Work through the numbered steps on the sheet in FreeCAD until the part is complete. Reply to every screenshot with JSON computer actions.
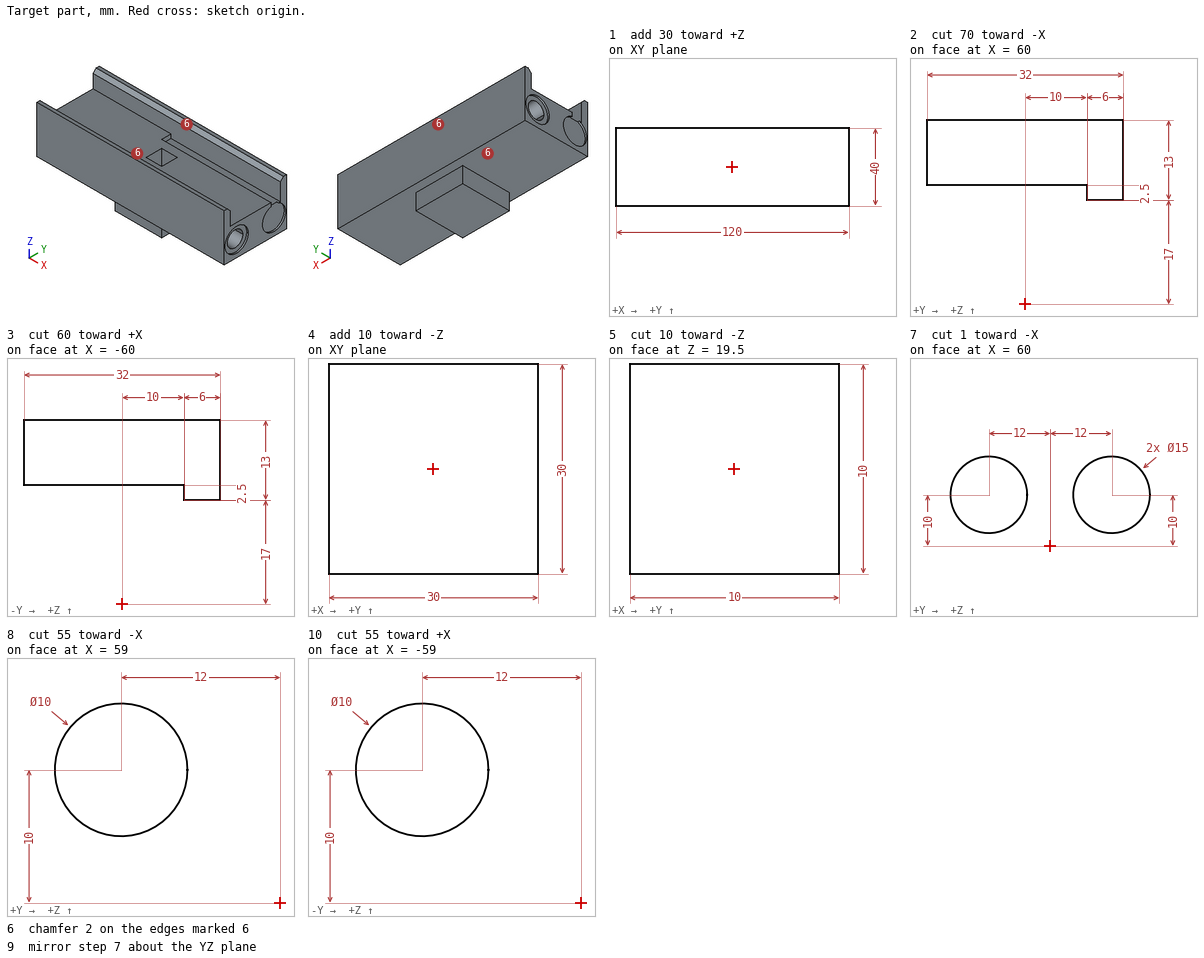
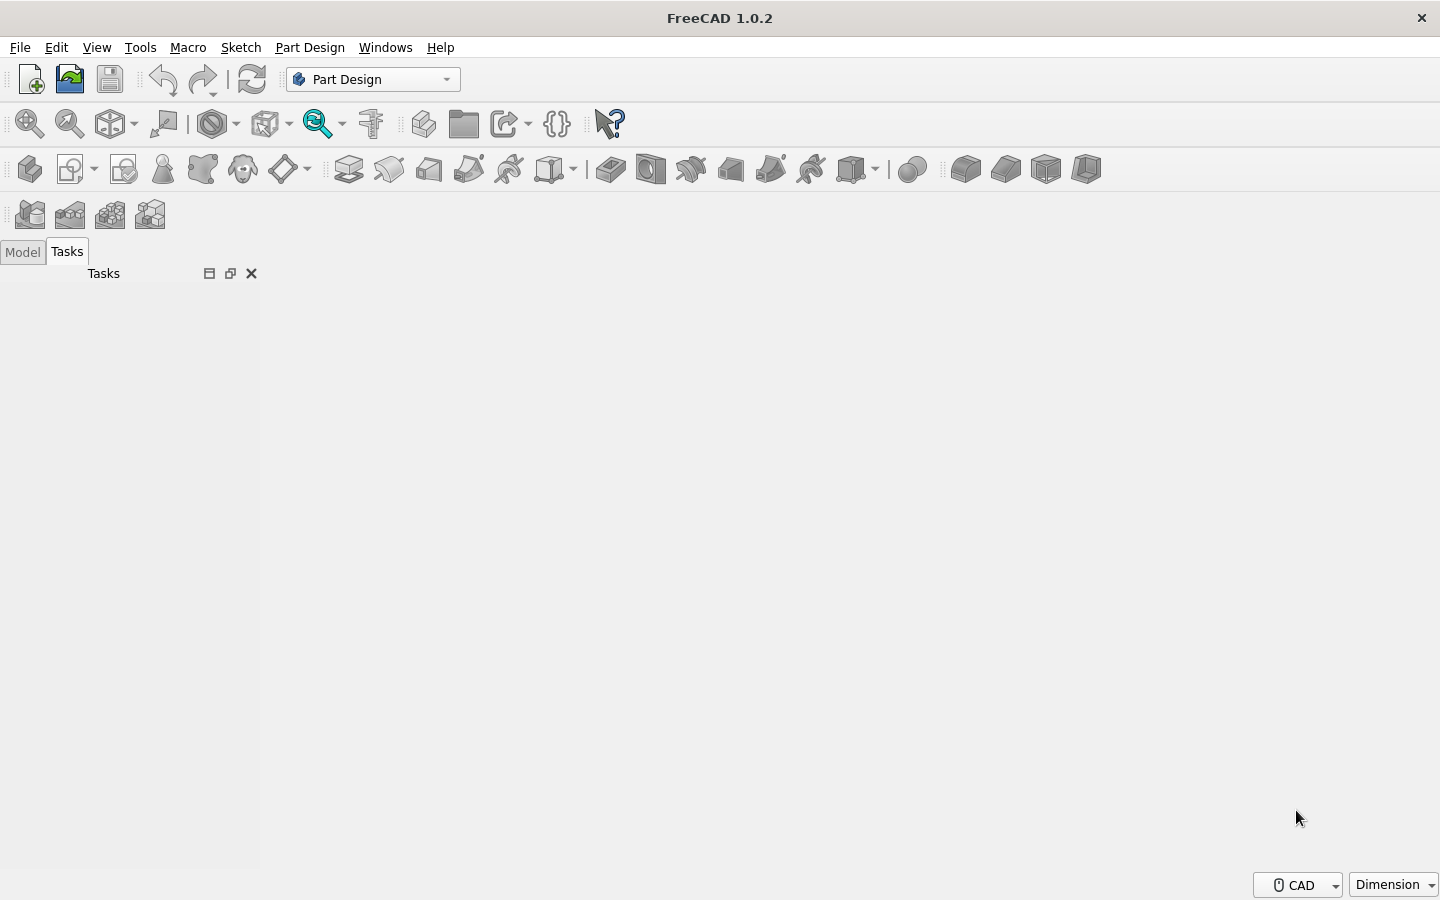
{"action": "key", "text": "ctrl+n"}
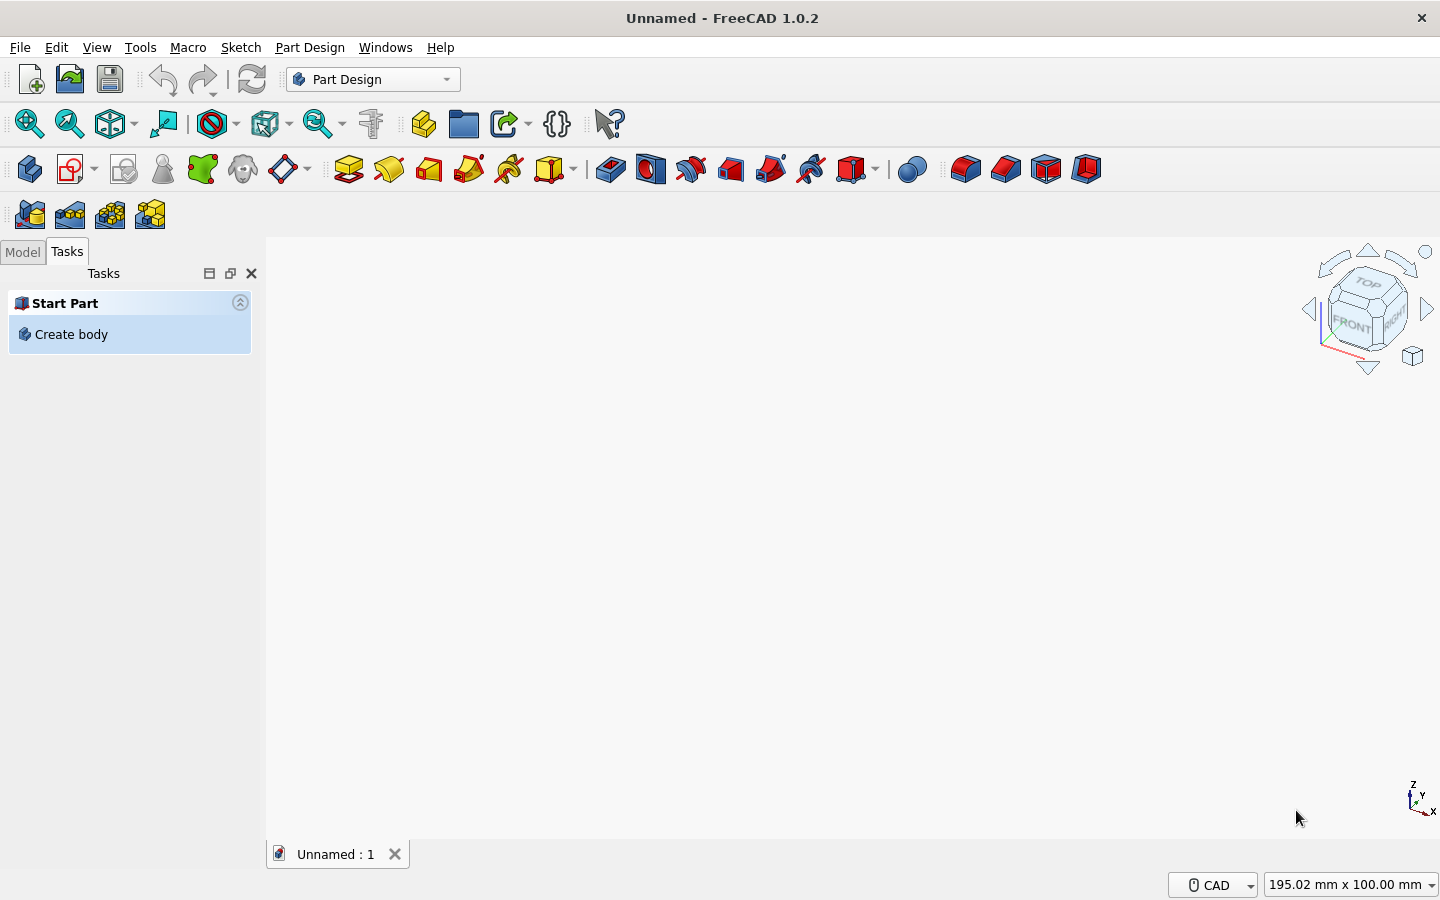
{"action": "left_click", "coordinate": [70, 170]}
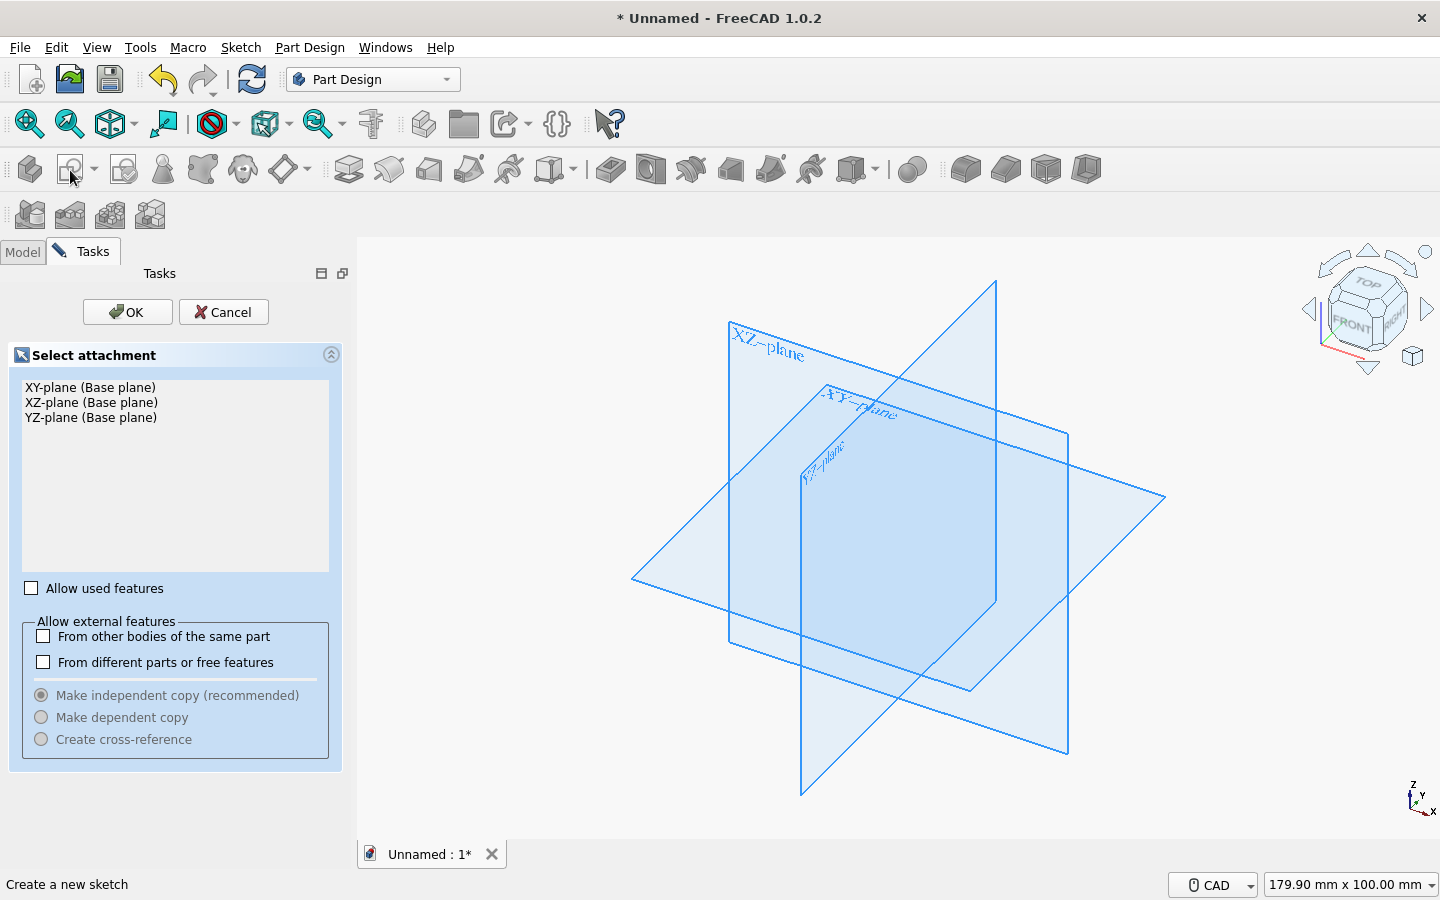
{"action": "left_click", "coordinate": [82, 388]}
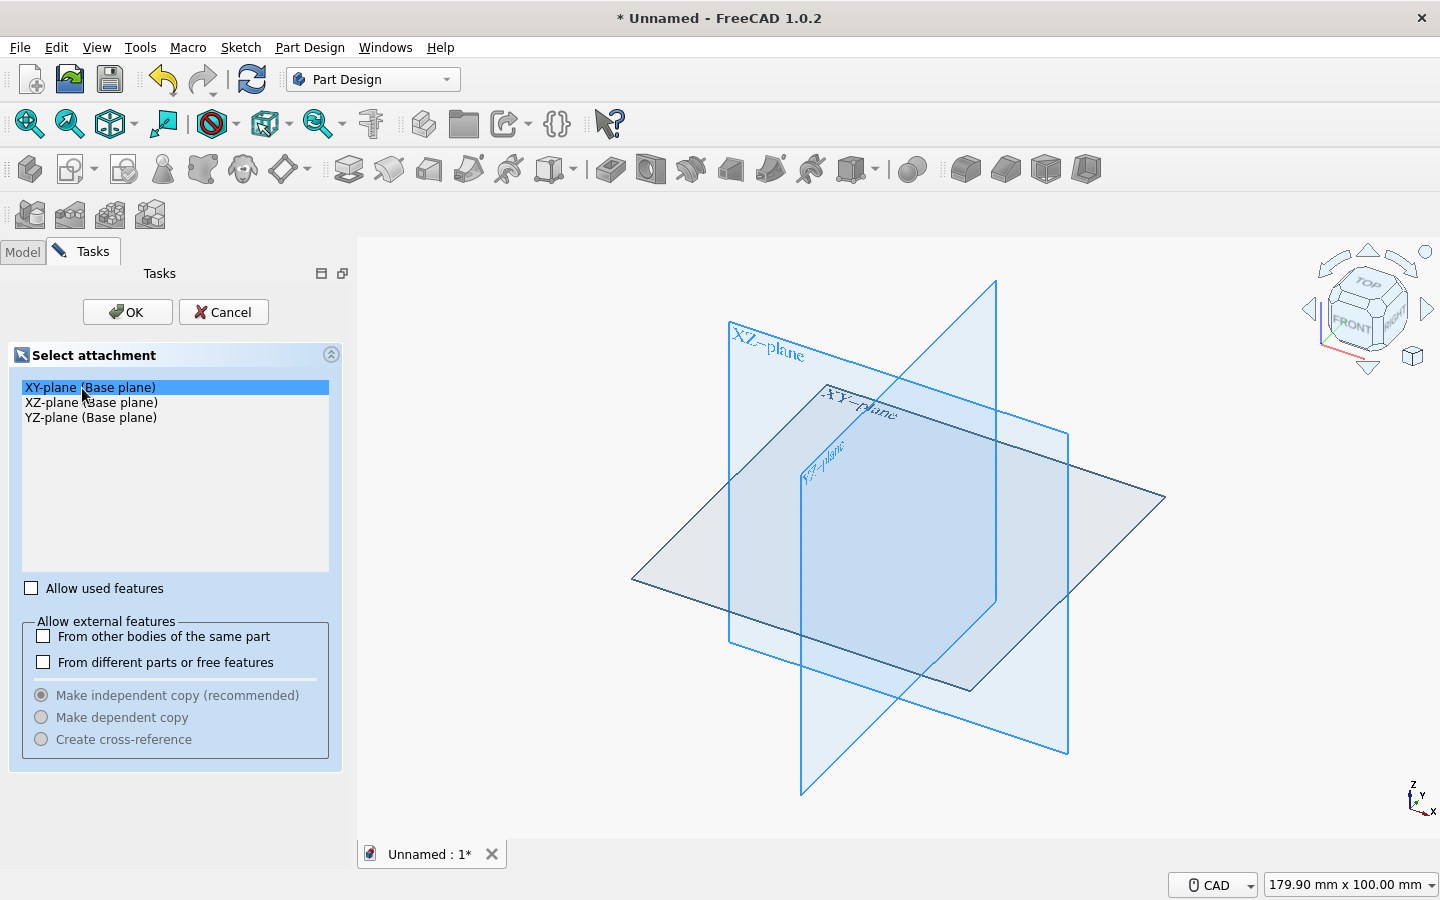
{"action": "left_click", "coordinate": [128, 312]}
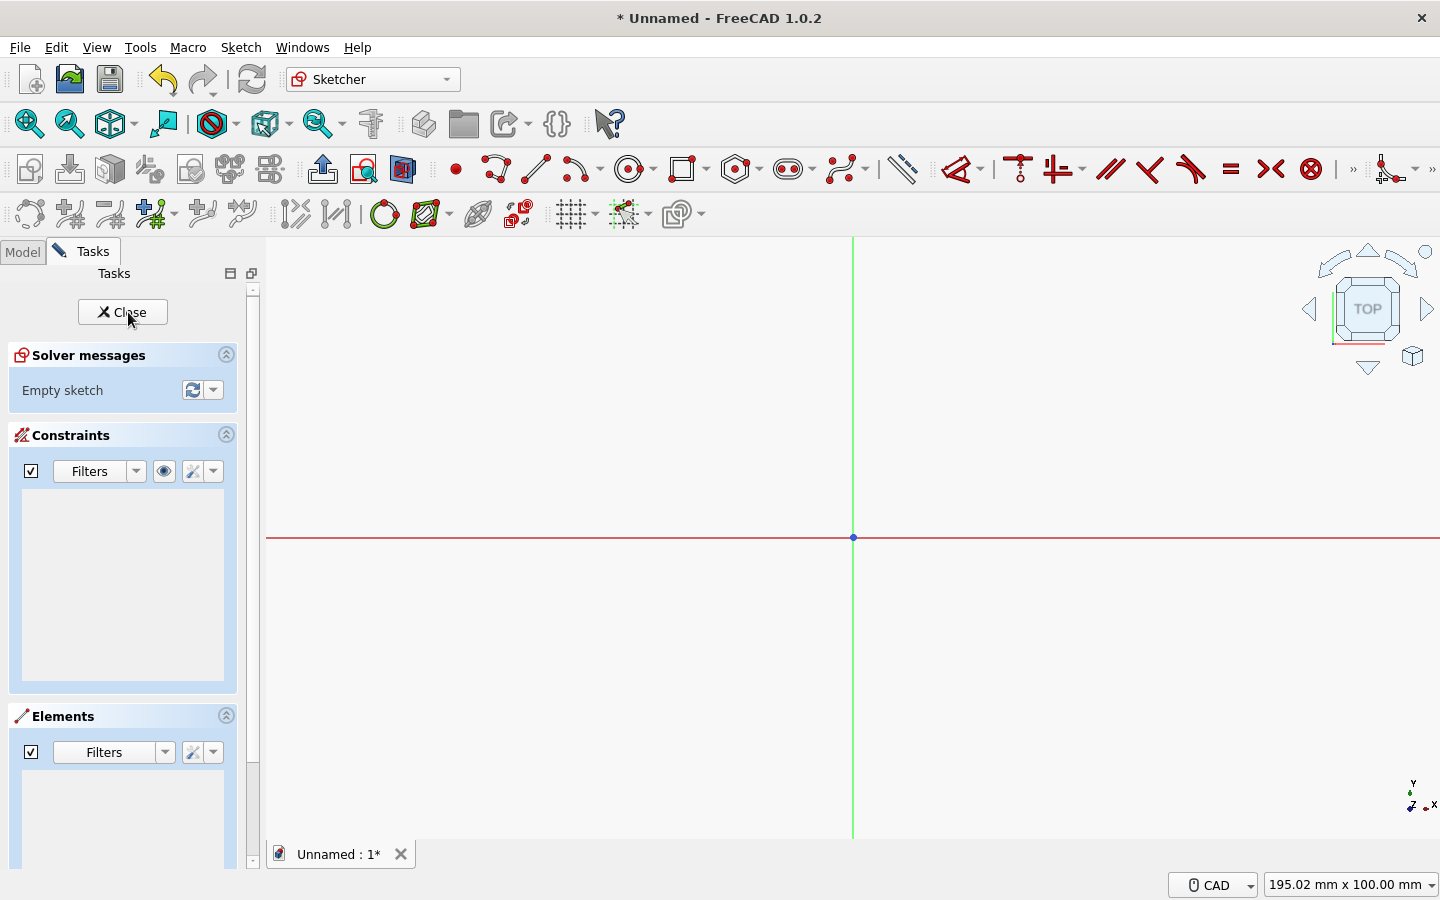
{"action": "key", "text": "g v"}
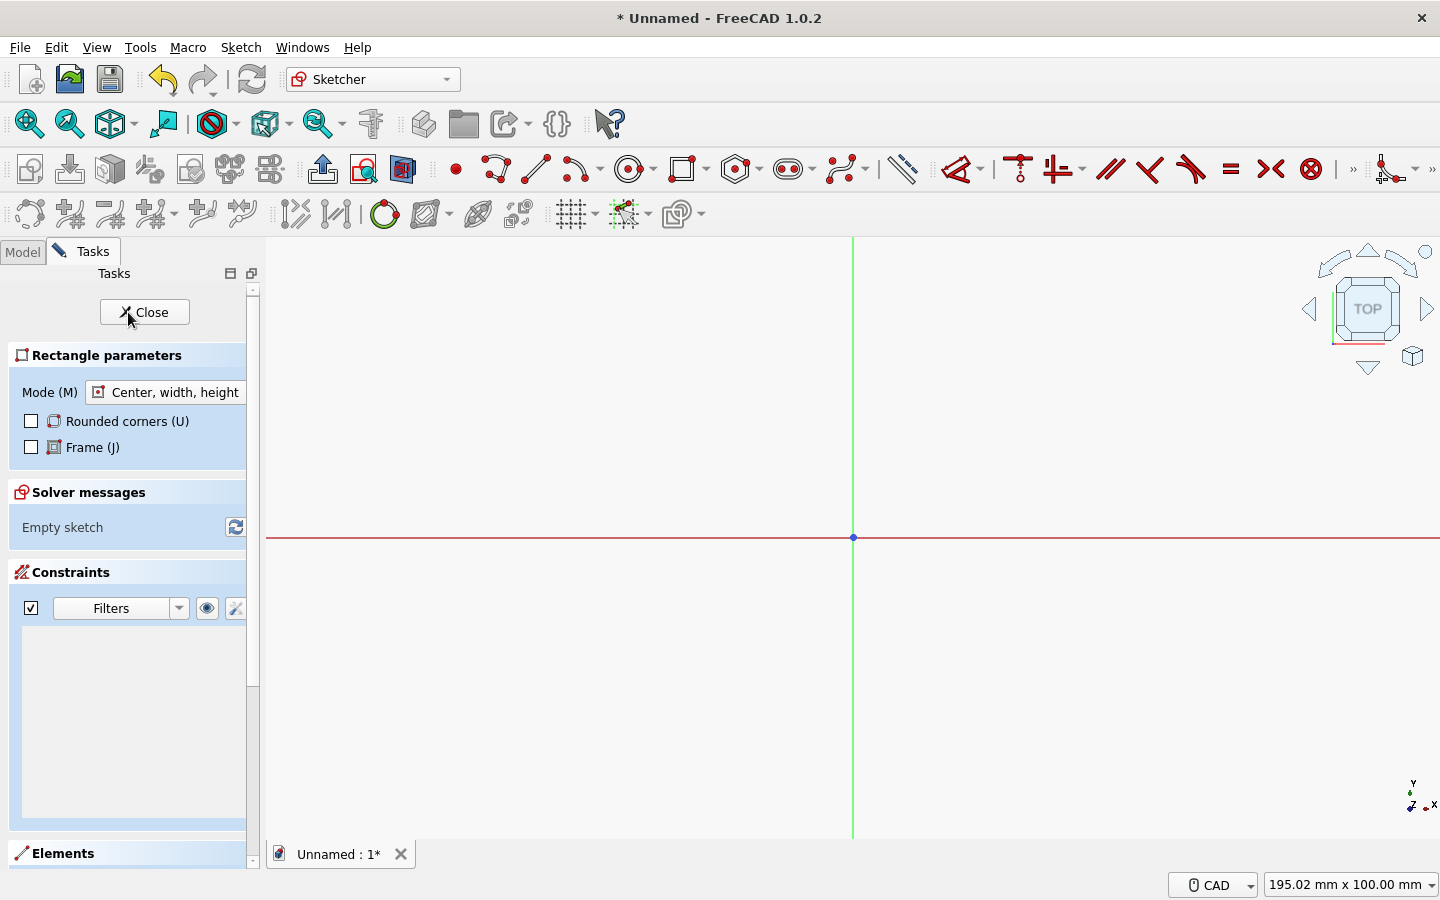
{"action": "left_click", "coordinate": [853, 538]}
{"action": "mouse_move", "coordinate": [1214, 418]}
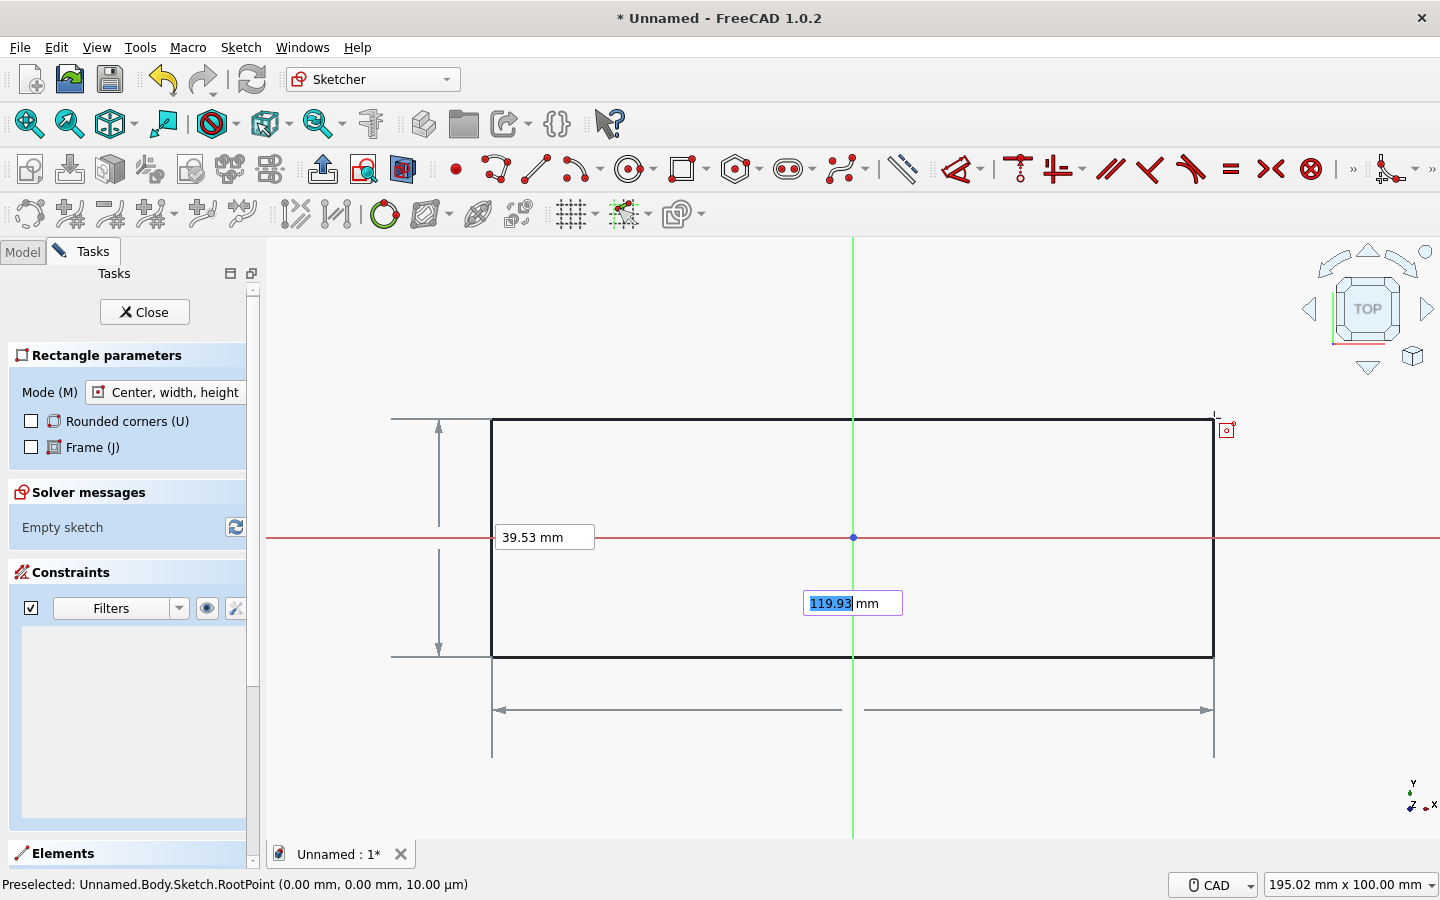
{"action": "type", "text": "120"}
{"action": "key", "text": "Tab"}
{"action": "type", "text": "40"}
{"action": "key", "text": "Return"}
{"action": "key", "text": "Escape"}